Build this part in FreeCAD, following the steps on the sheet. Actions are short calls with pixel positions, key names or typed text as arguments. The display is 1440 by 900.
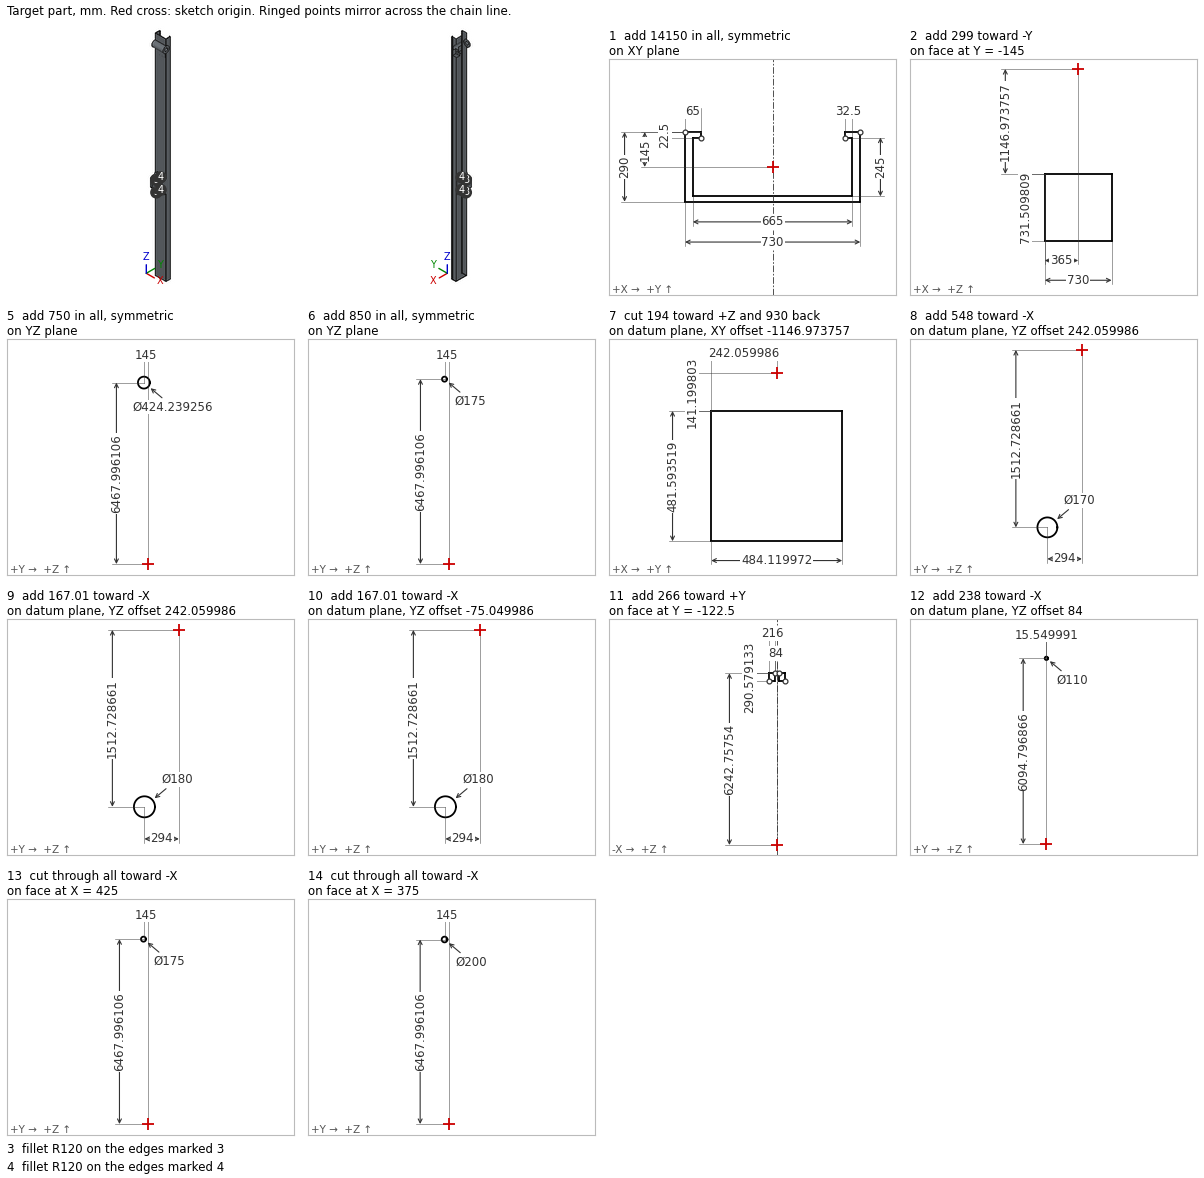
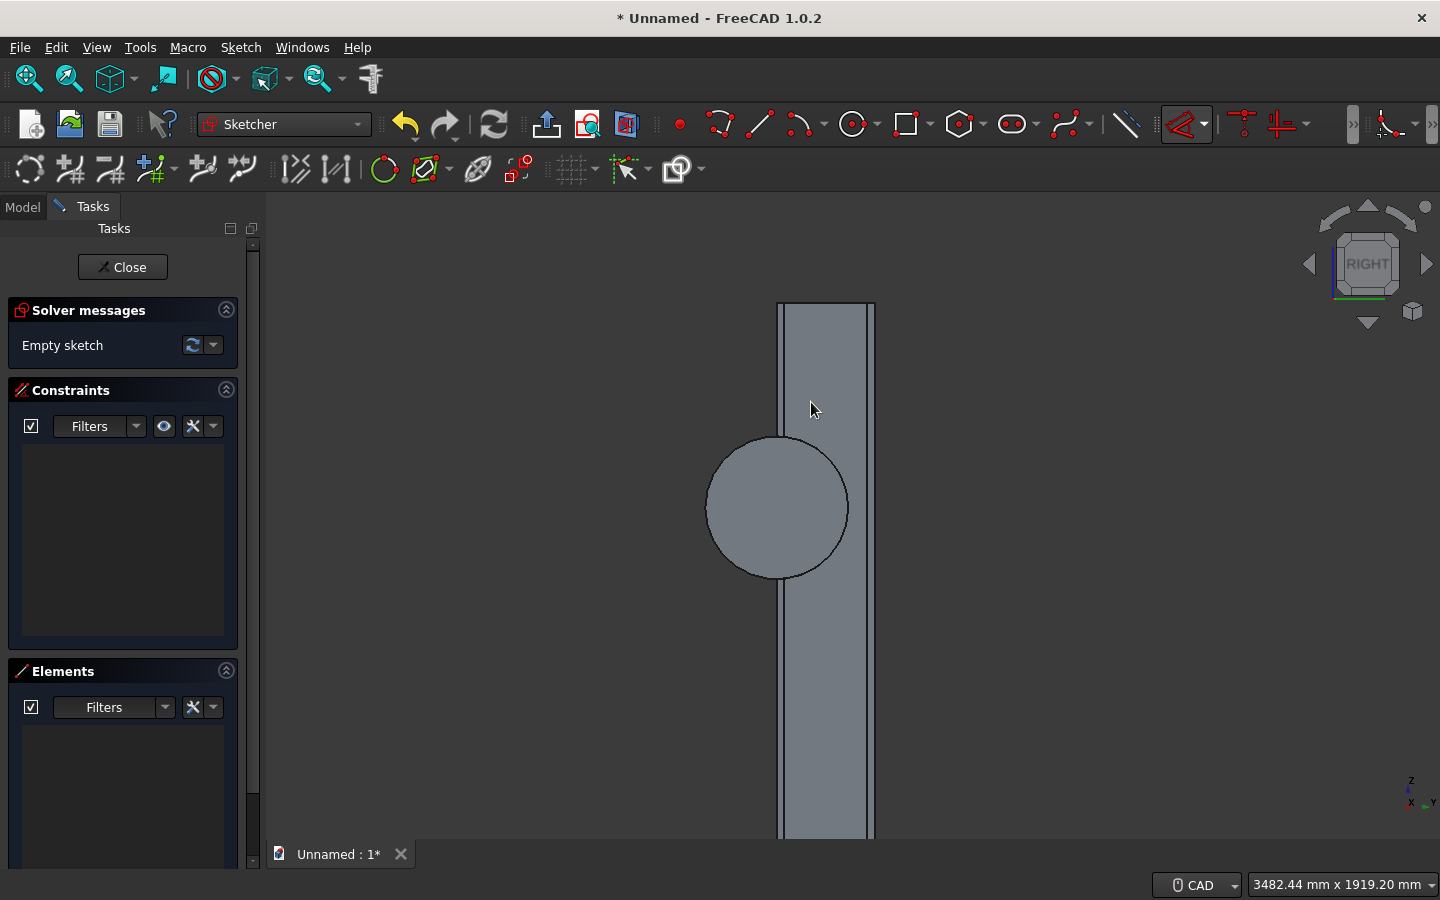
scroll(776, 507, up, 10)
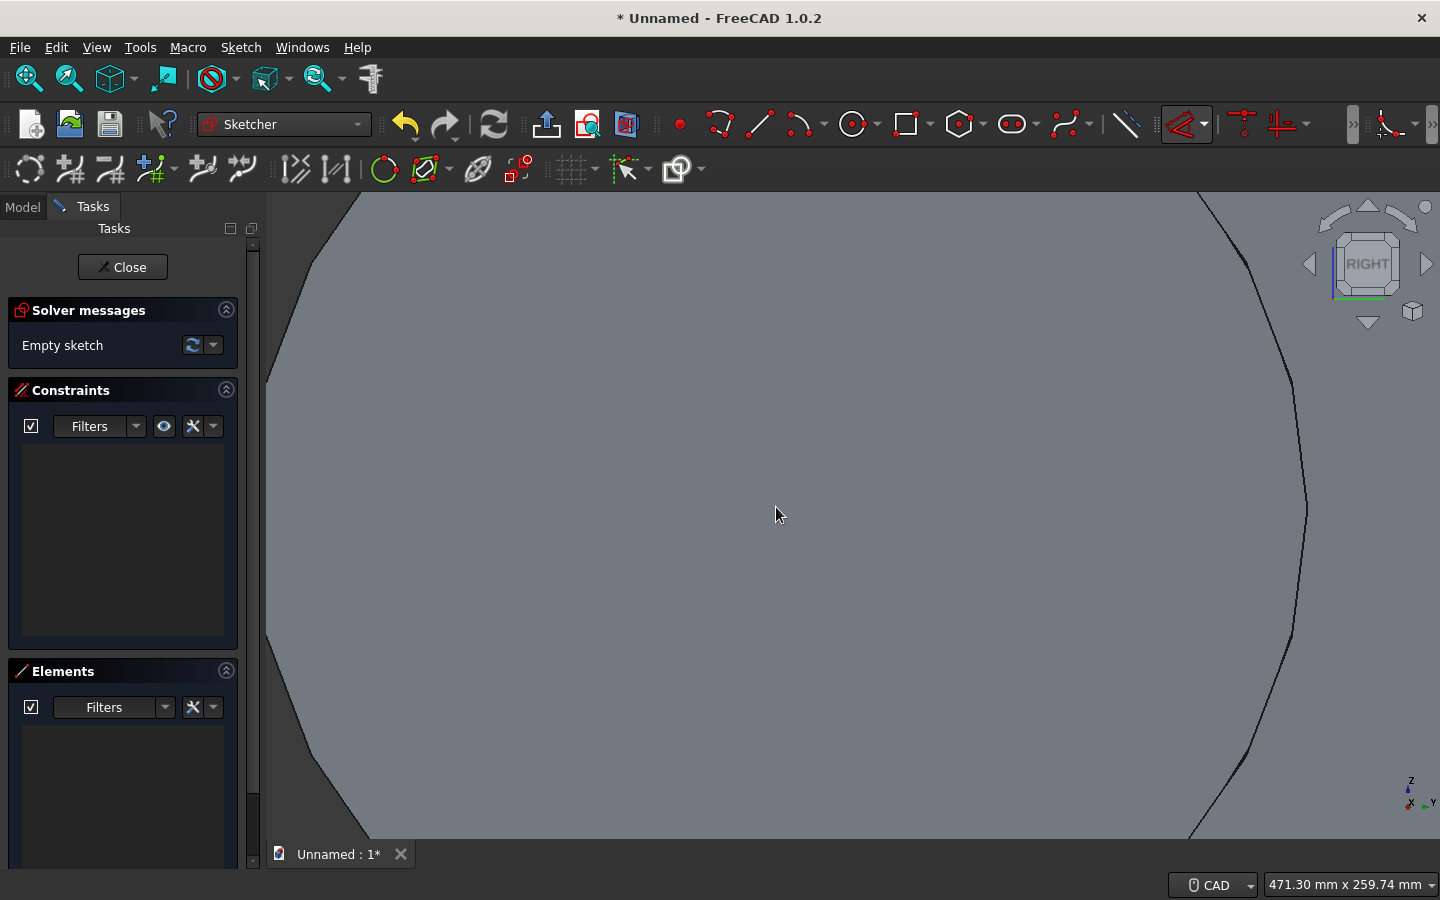
click(854, 124)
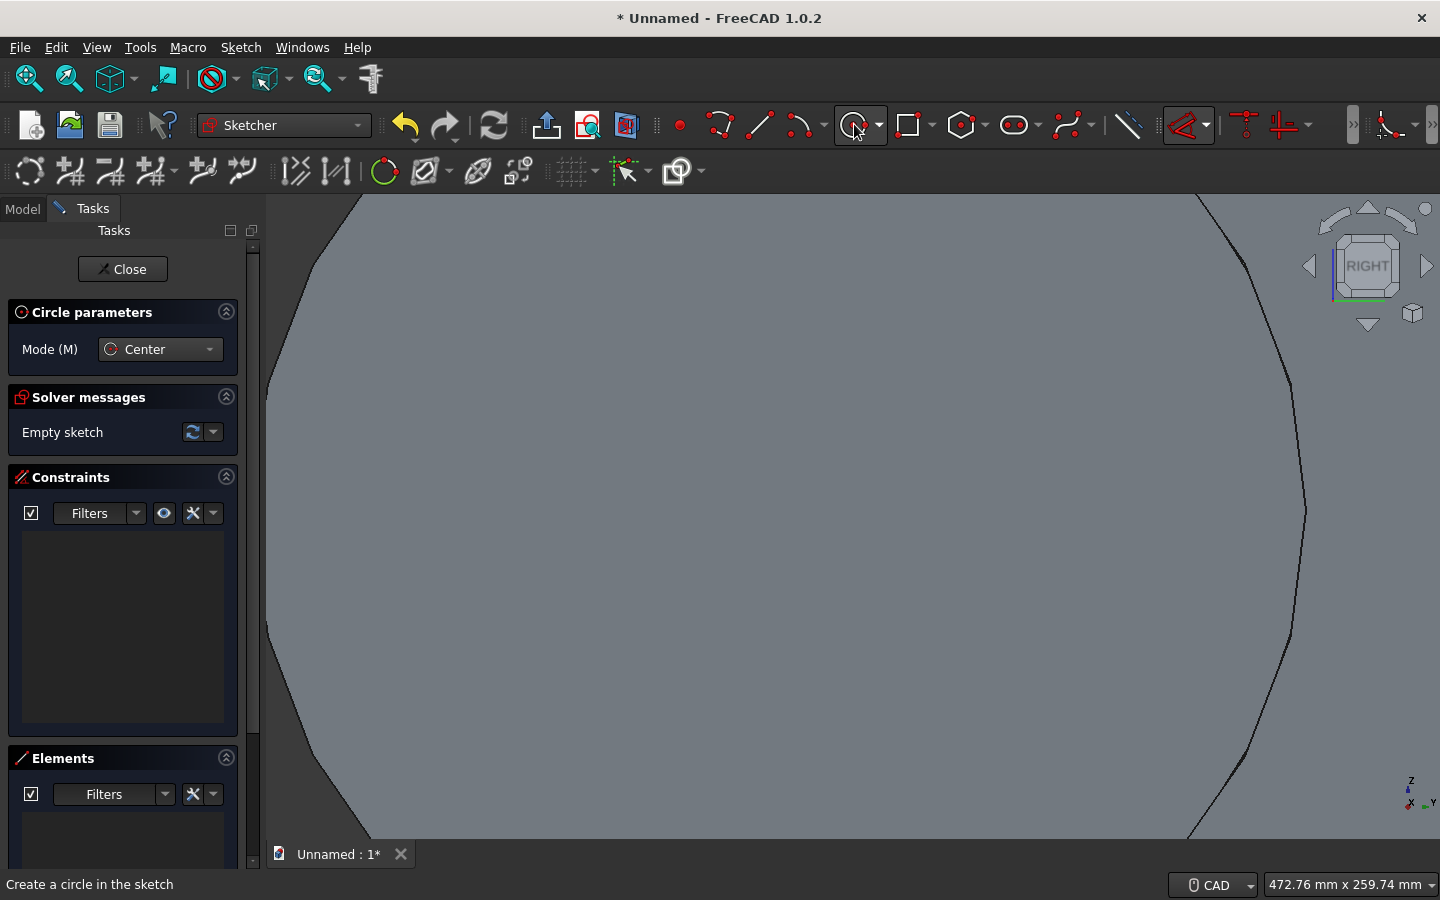
click(779, 510)
click(933, 357)
key(Escape)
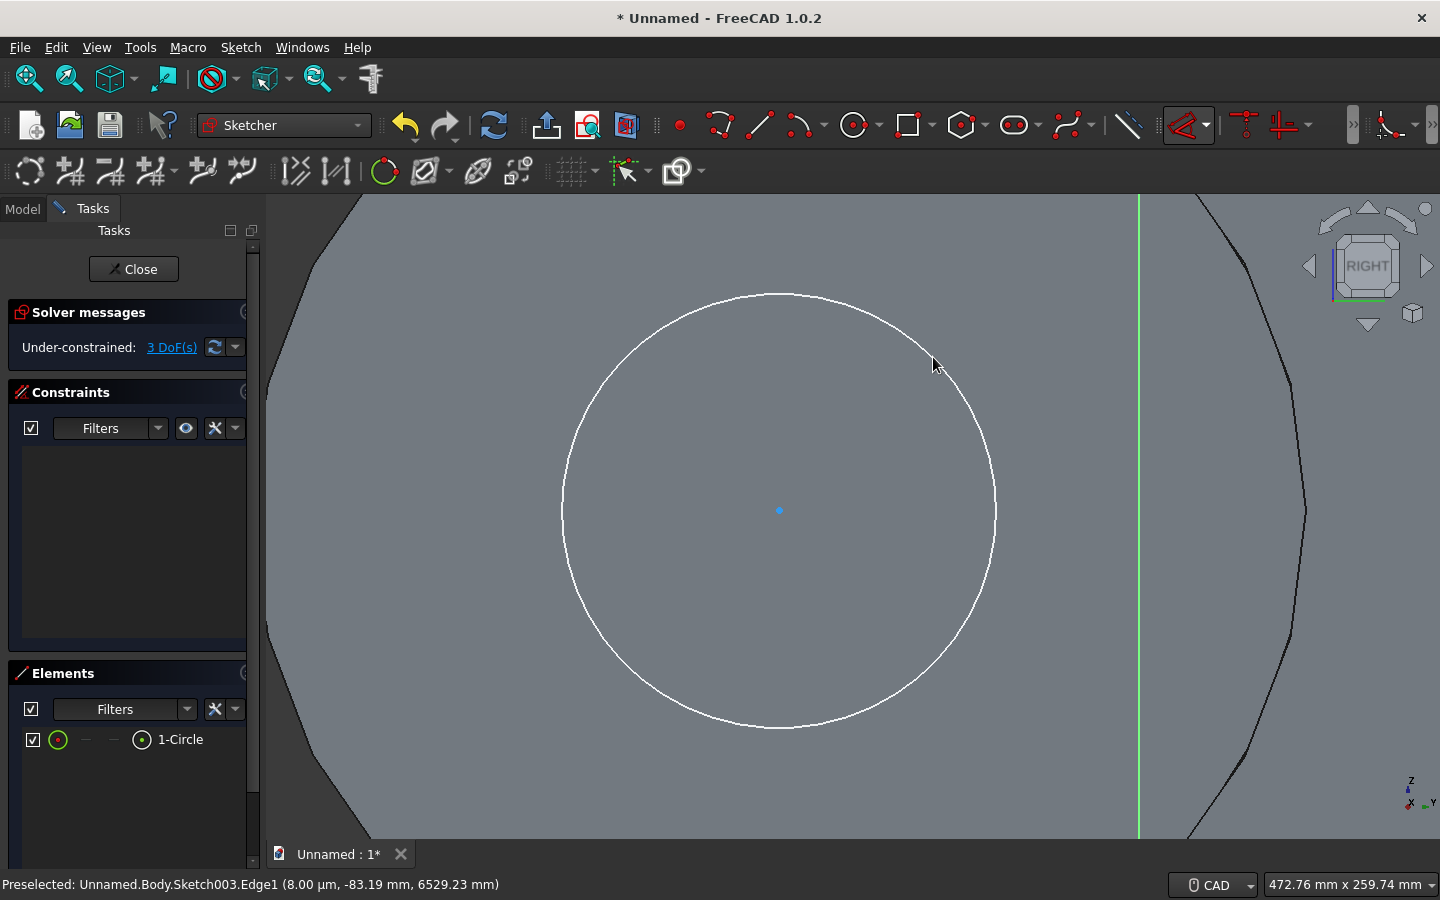
click(932, 357)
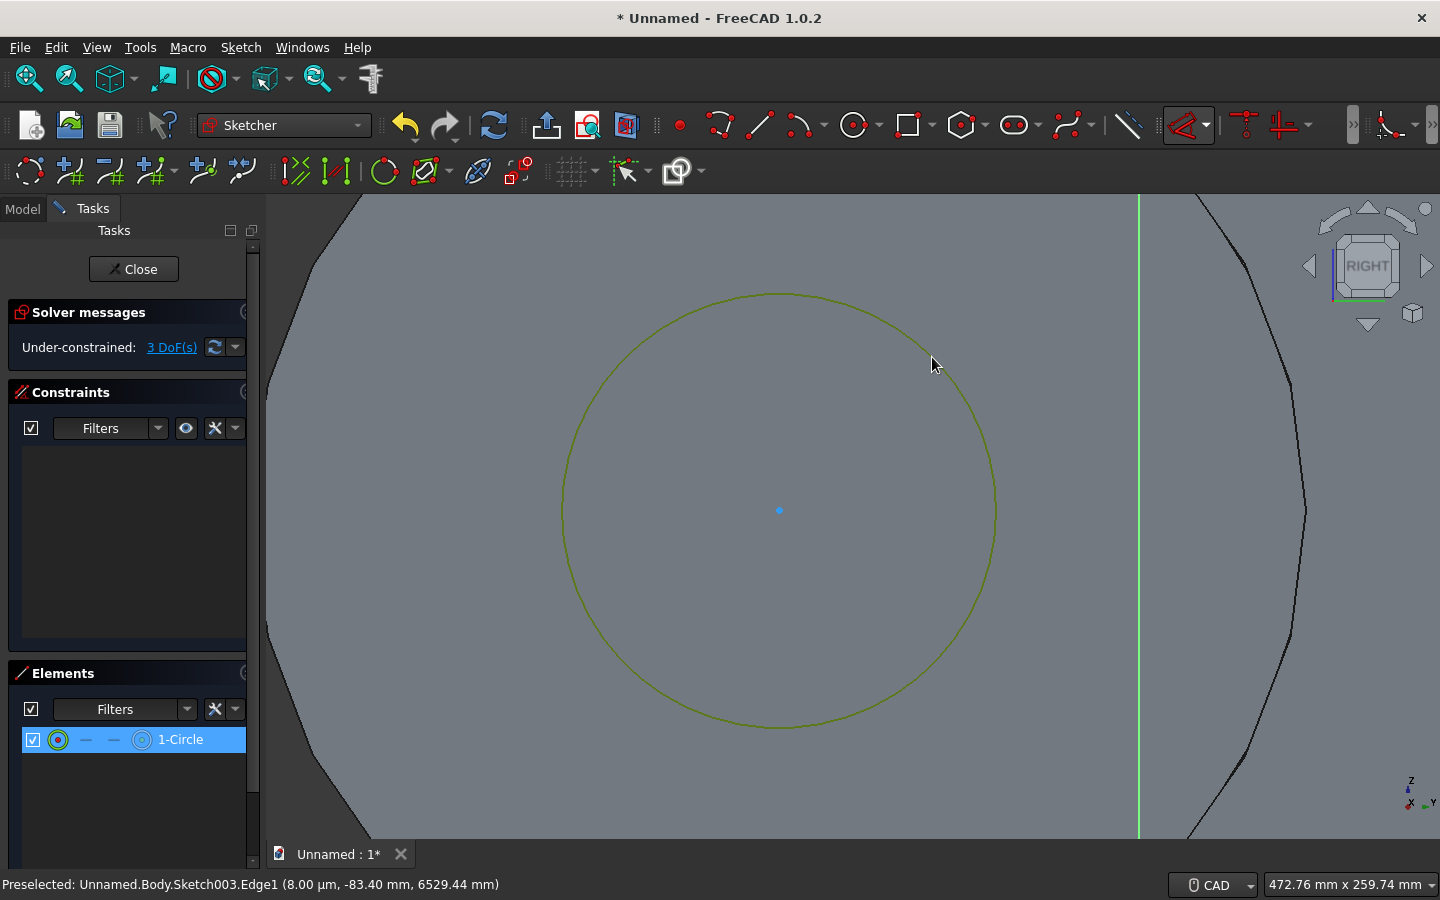
click(1208, 126)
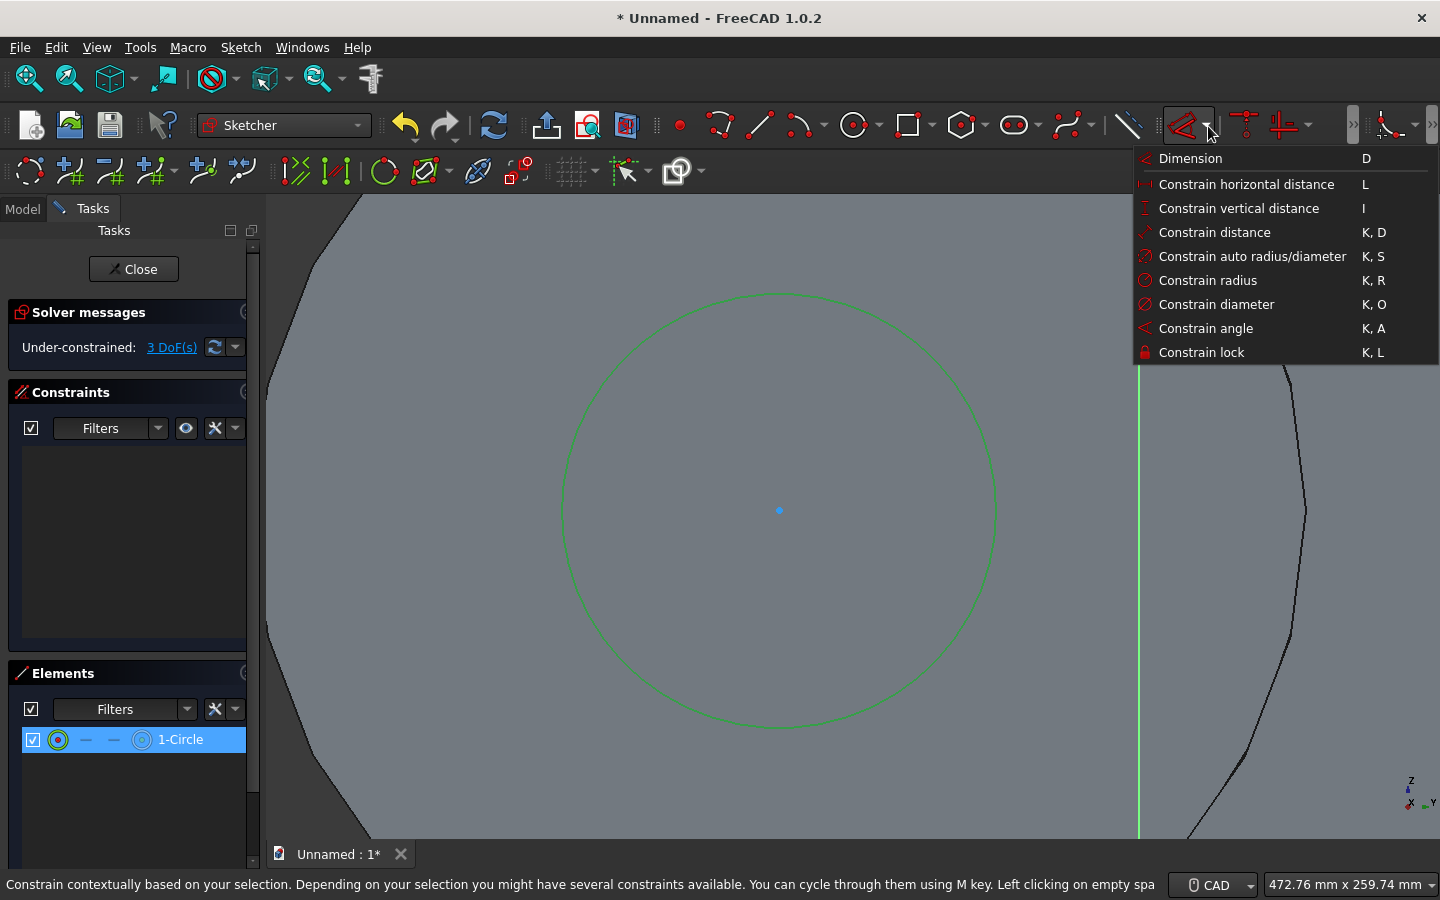
click(1286, 304)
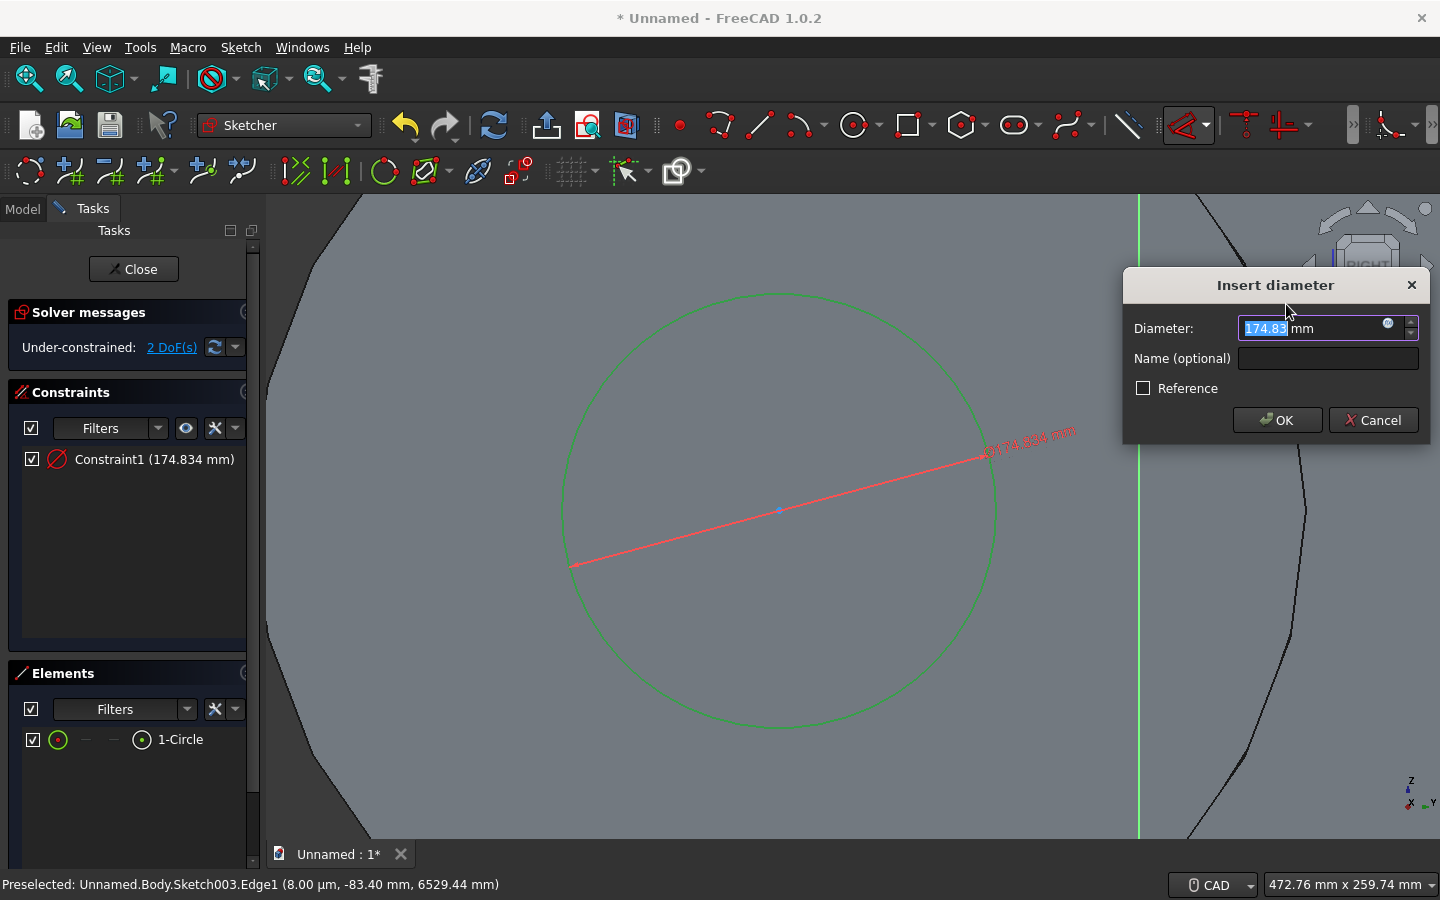
text(175)
key(Return)